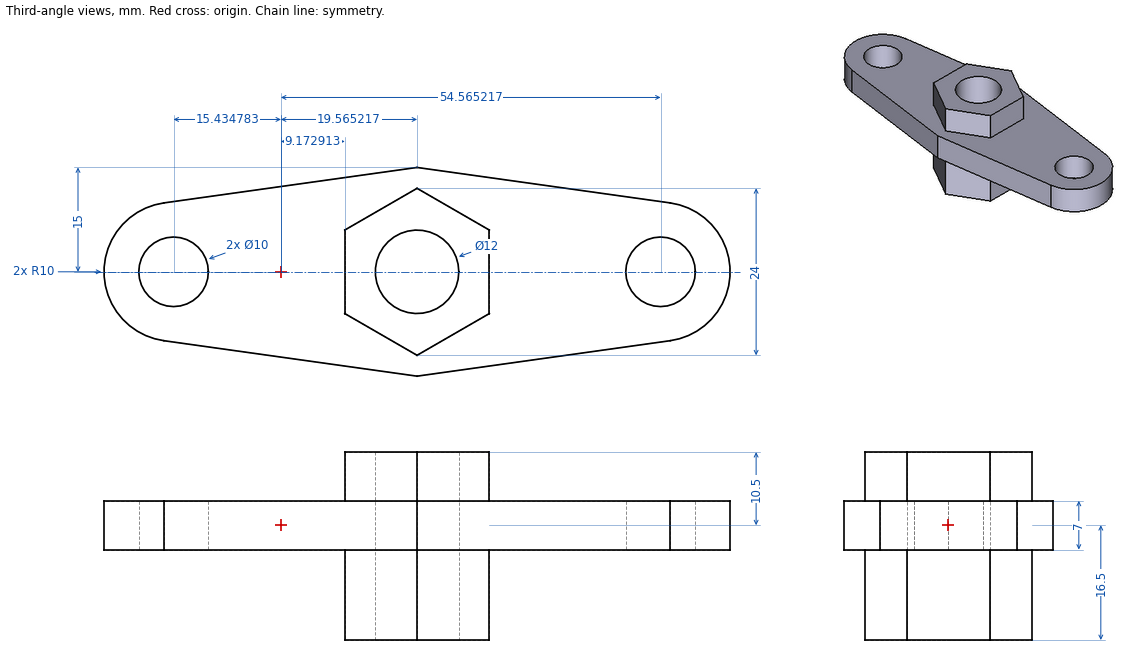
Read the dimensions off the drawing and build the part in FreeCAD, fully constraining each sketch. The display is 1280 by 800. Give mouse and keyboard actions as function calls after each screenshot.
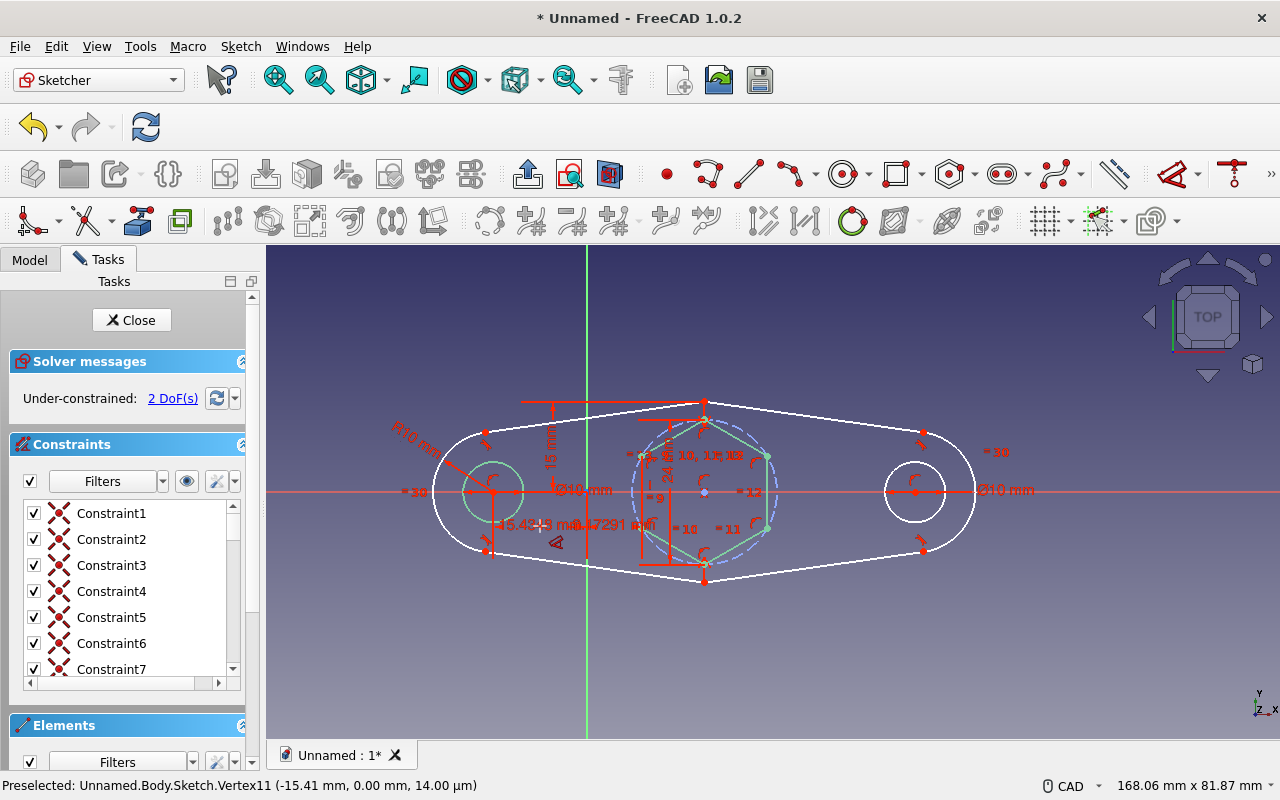
click(915, 492)
click(826, 526)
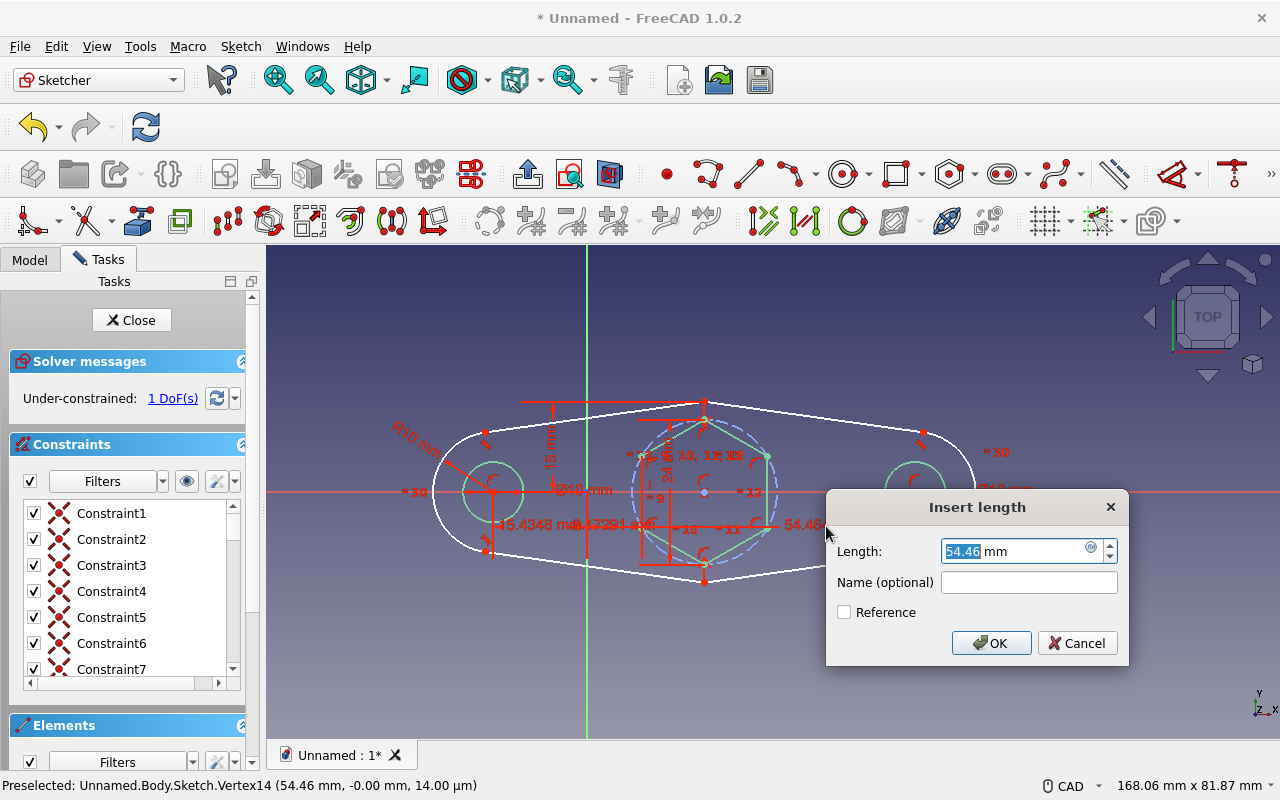
text(54.565217)
key(Return)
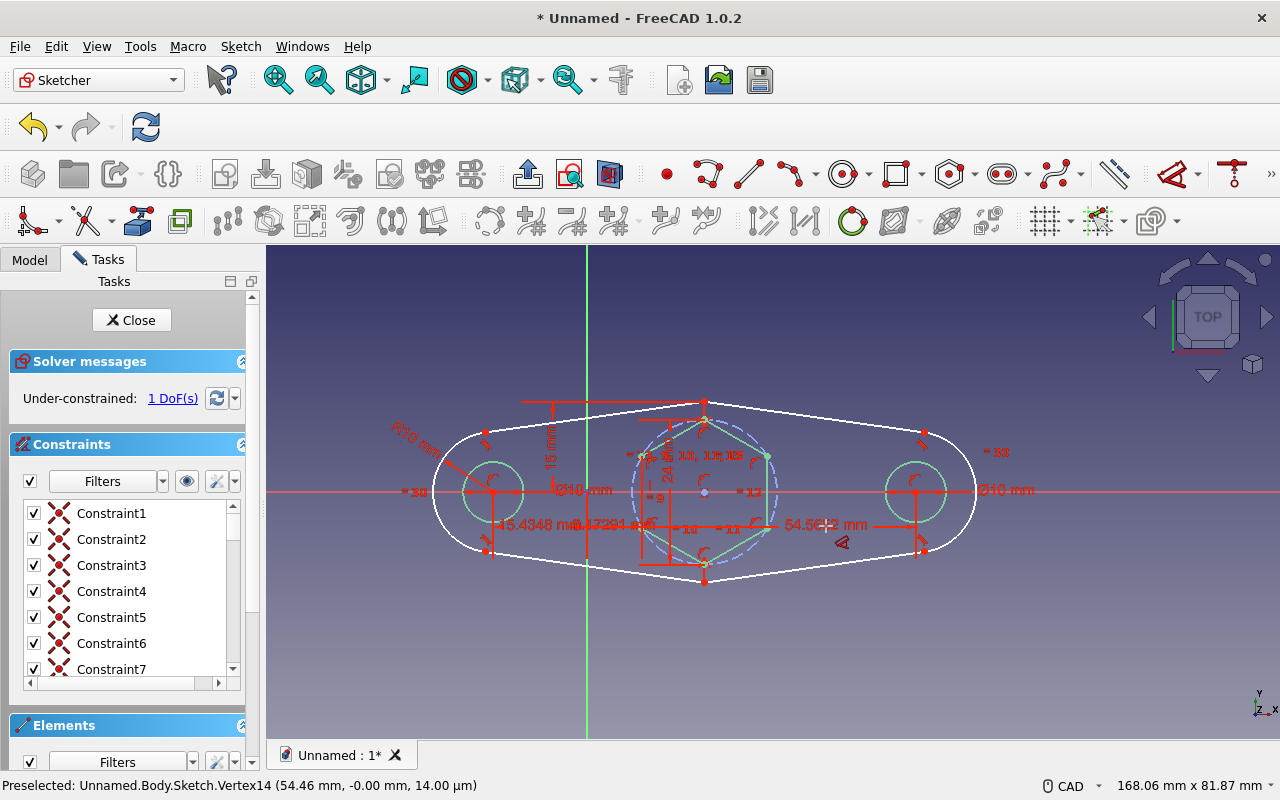
click(704, 402)
click(645, 368)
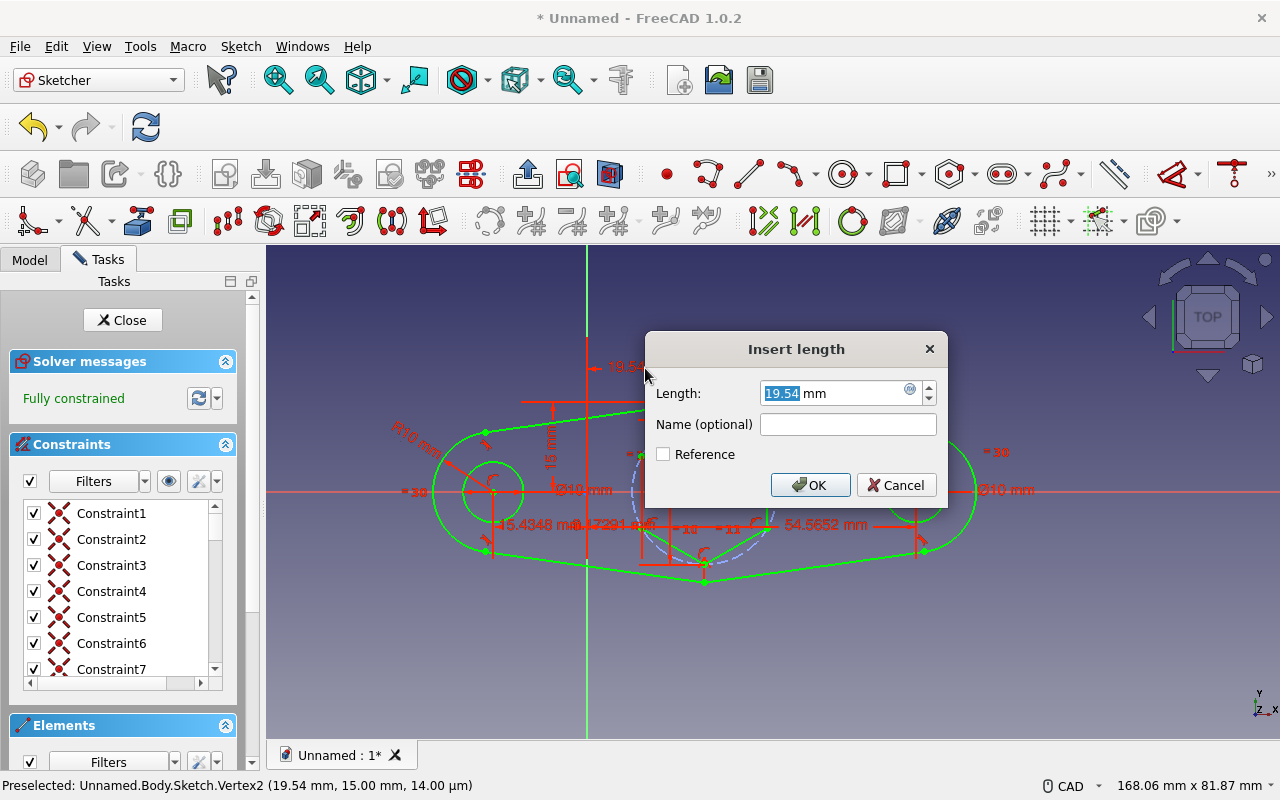
text(19.565217)
key(Return)
key(Escape)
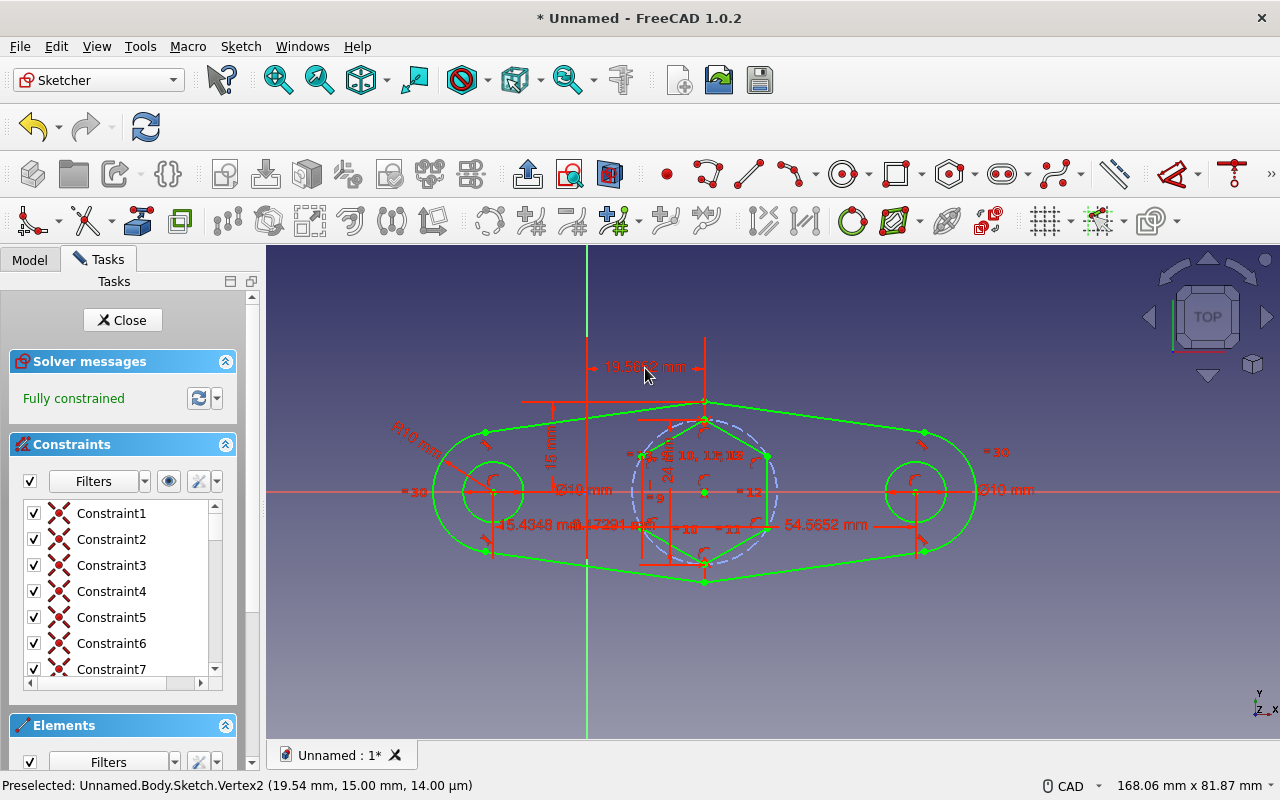
click(123, 320)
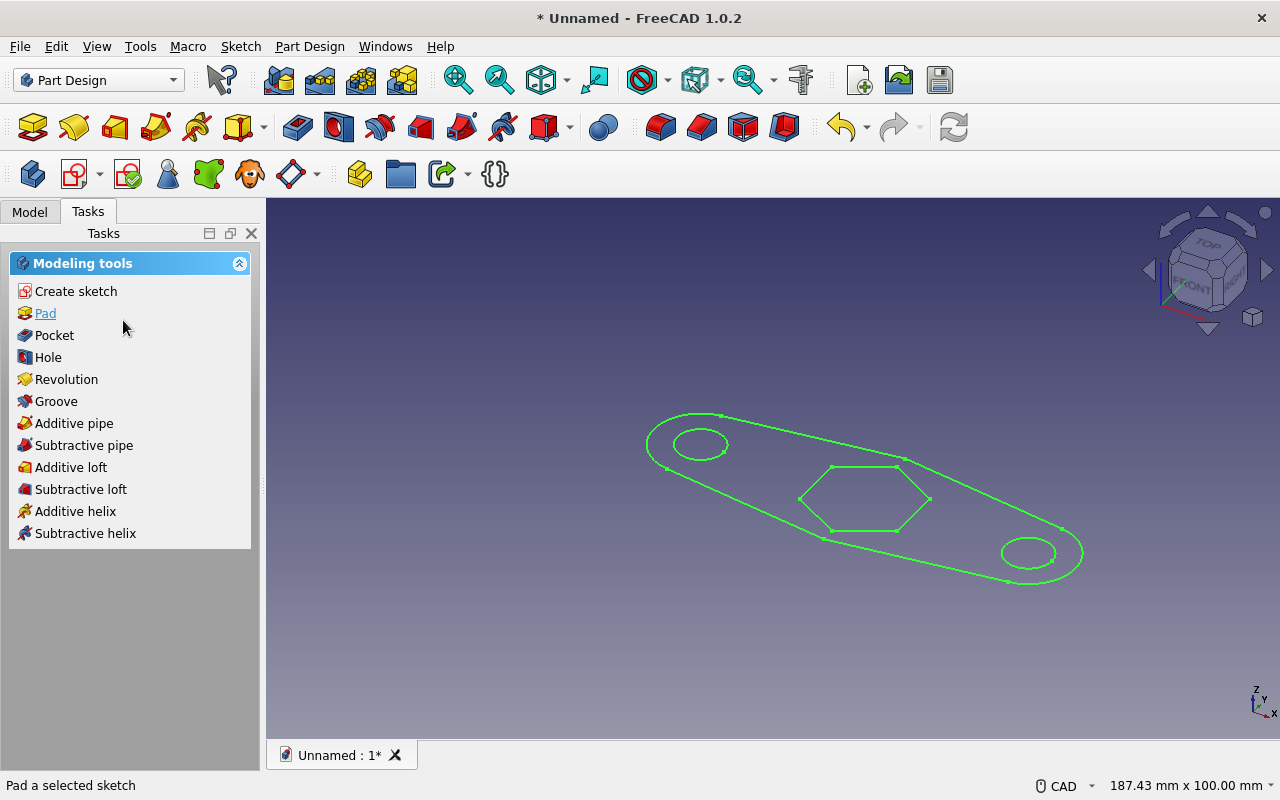
click(33, 128)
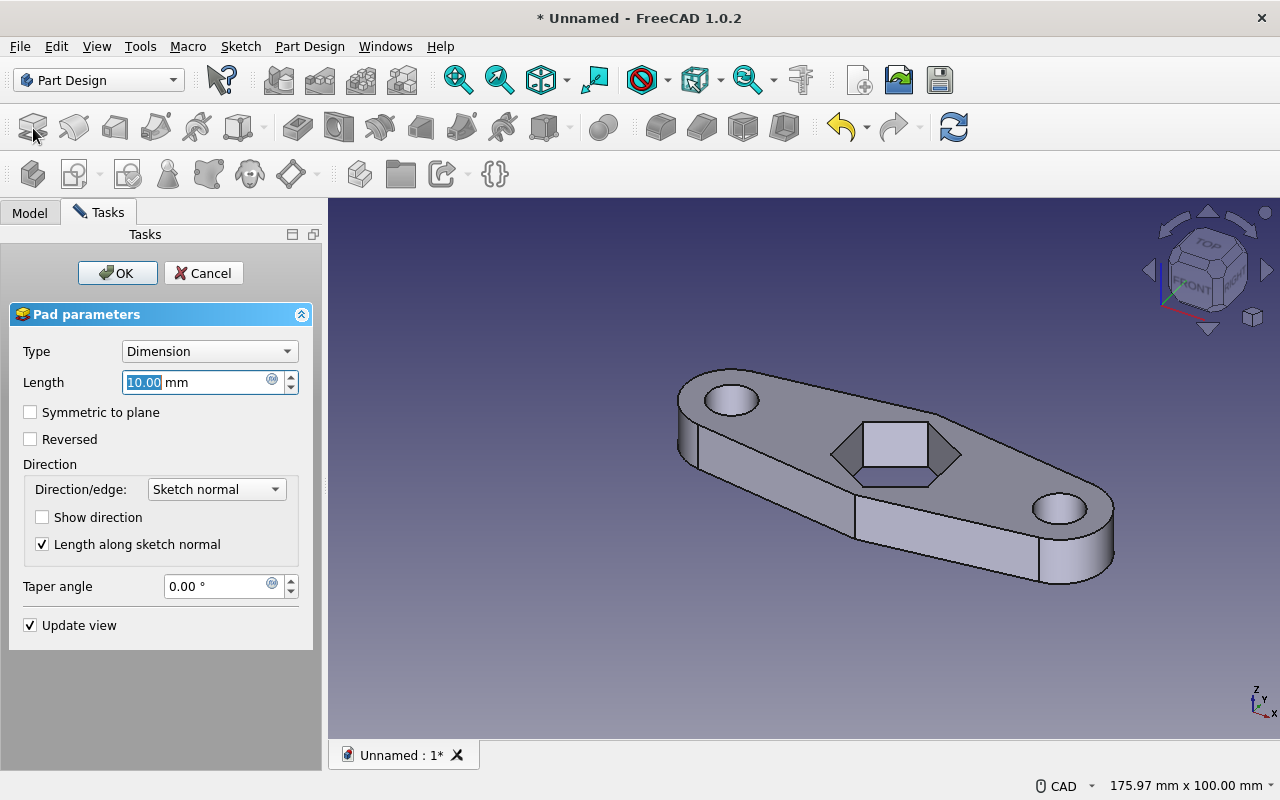
text(7)
key(Tab)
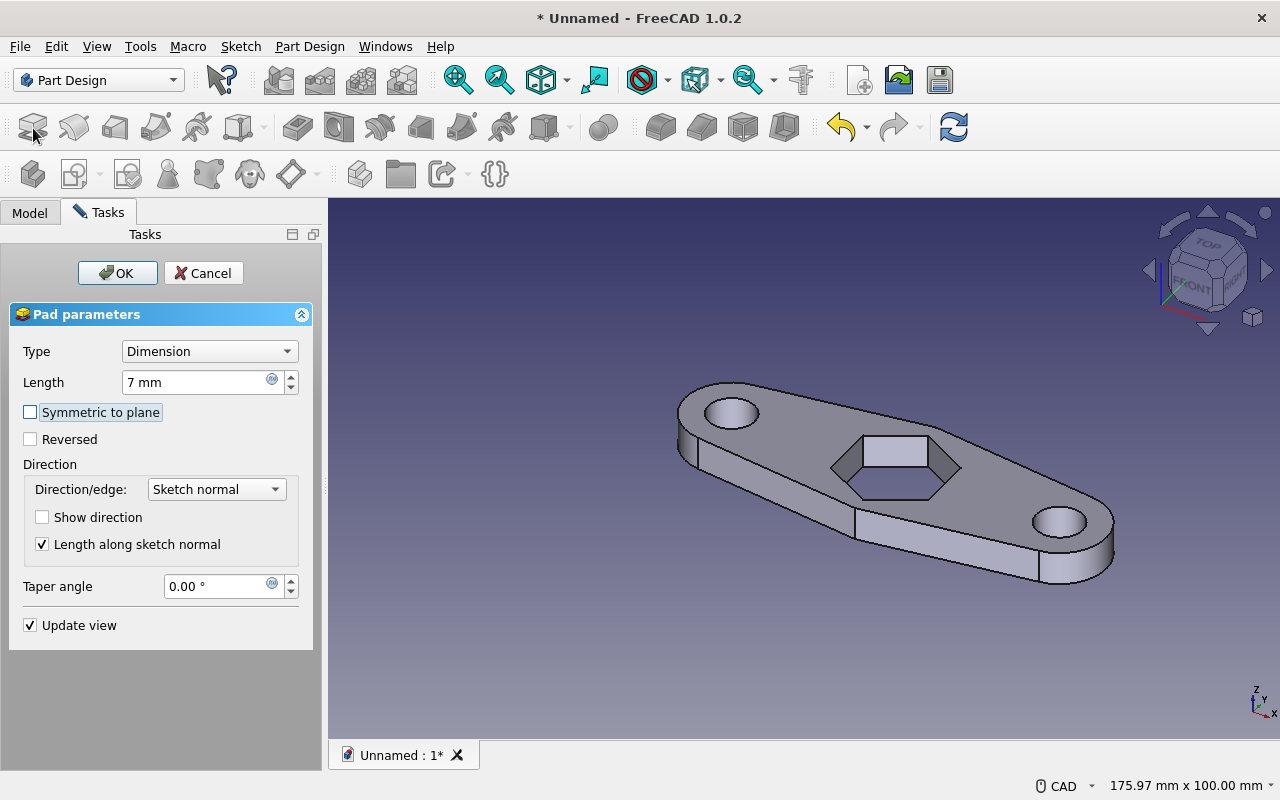
click(31, 412)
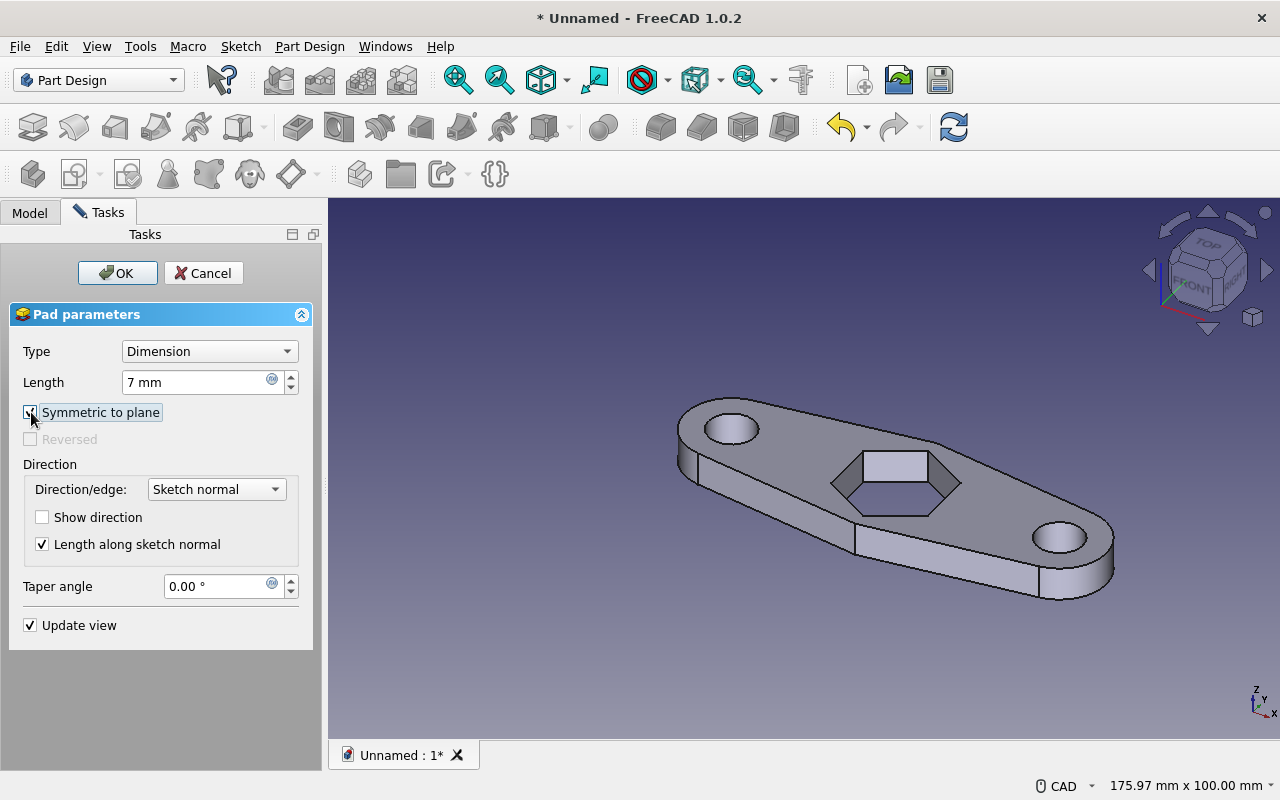
click(118, 273)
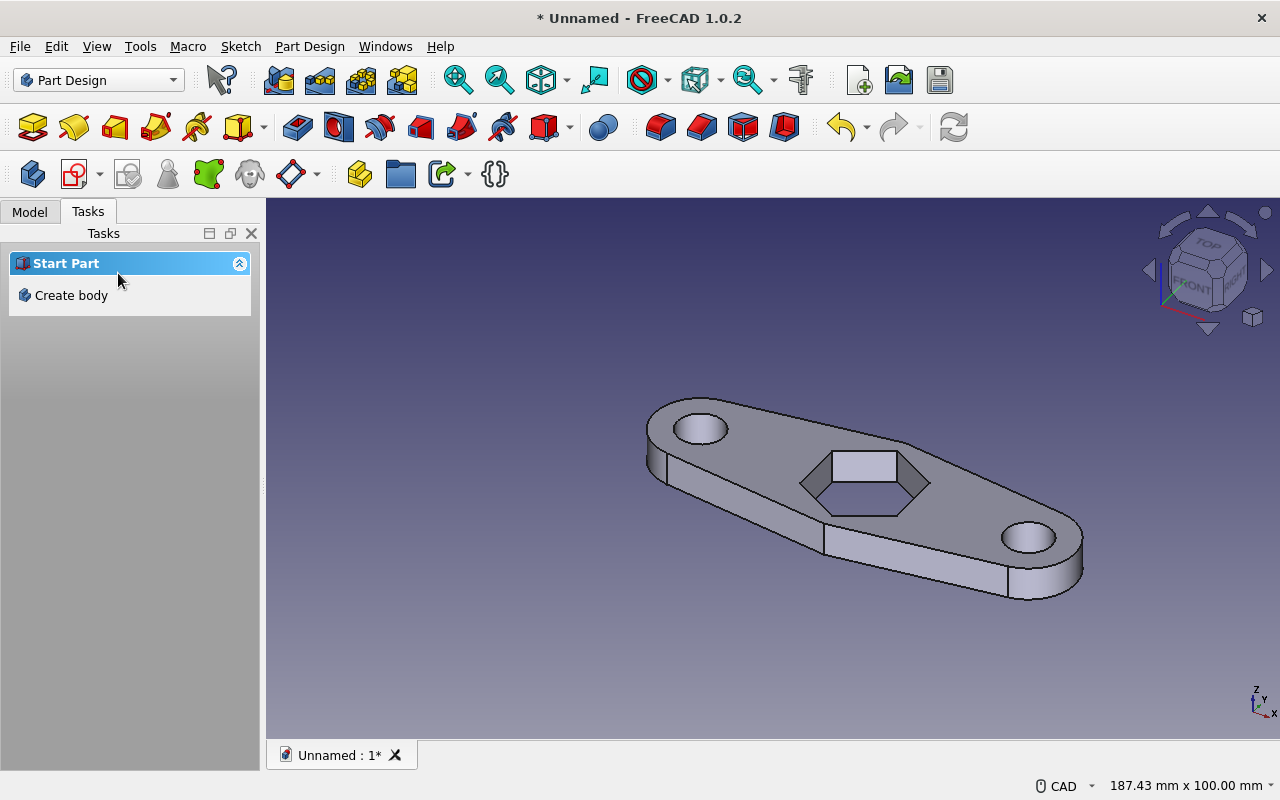
click(74, 174)